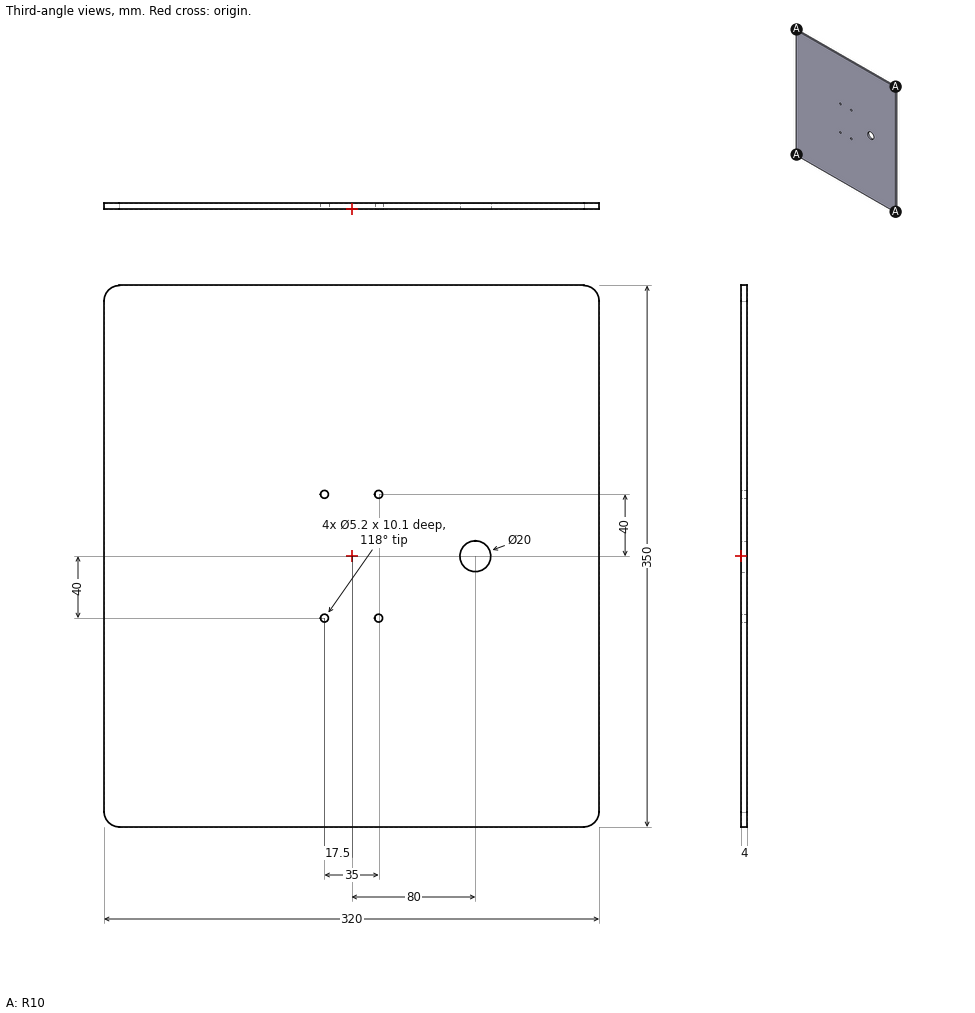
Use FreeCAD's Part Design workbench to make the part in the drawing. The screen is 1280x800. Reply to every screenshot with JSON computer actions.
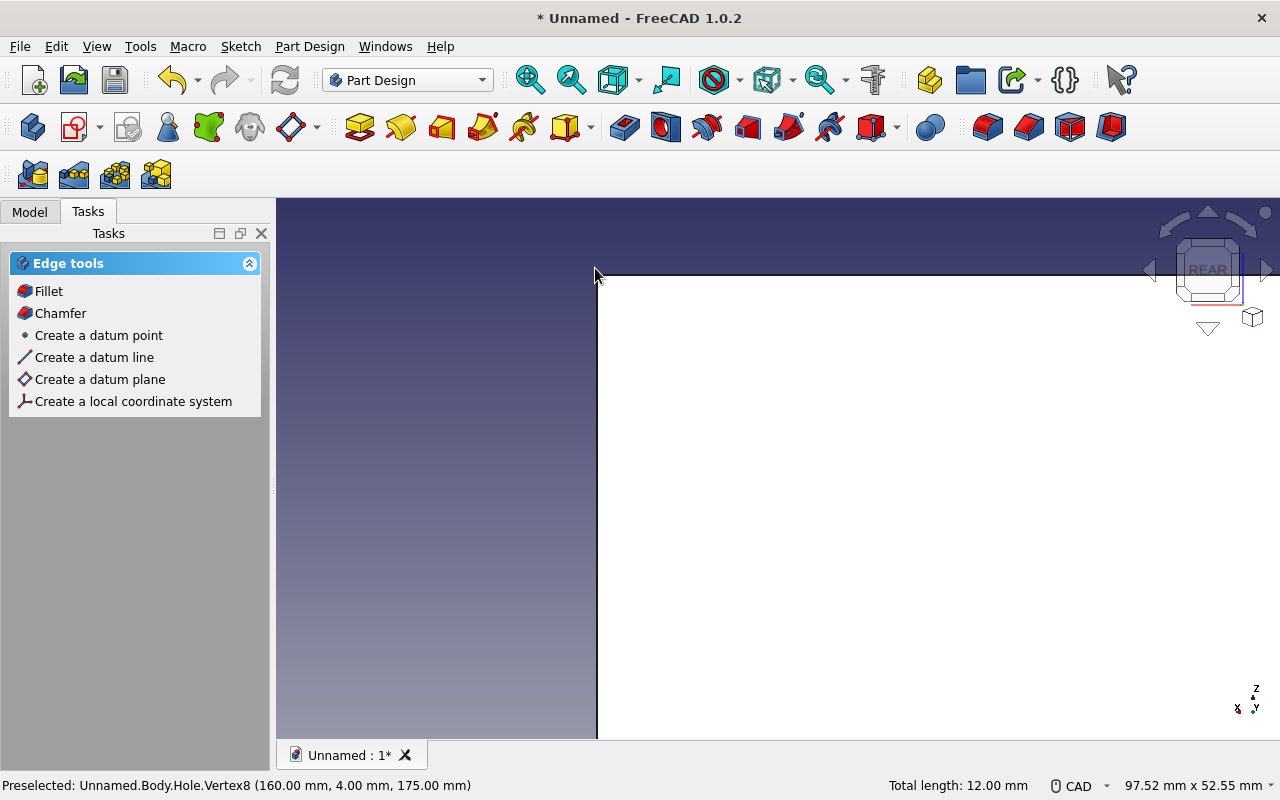
{"action": "key", "text": "v f"}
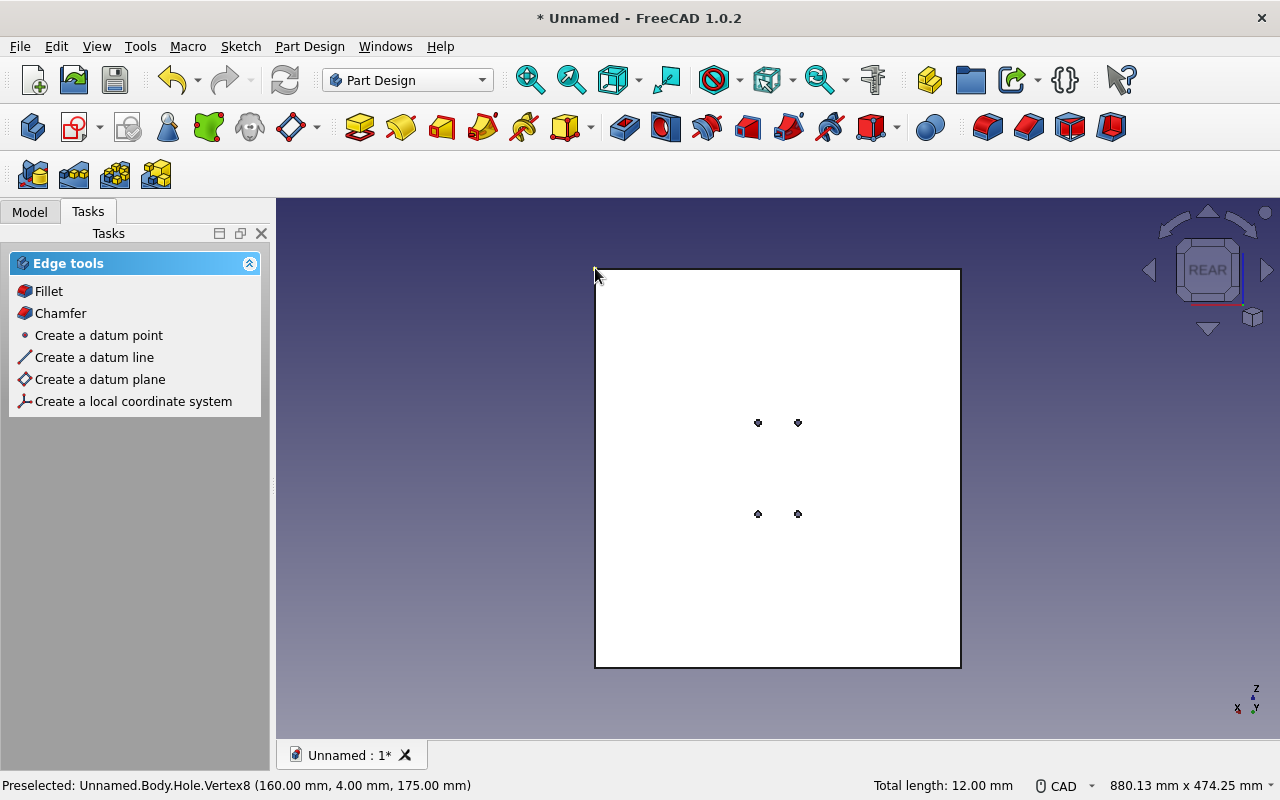
{"action": "key", "text": "6"}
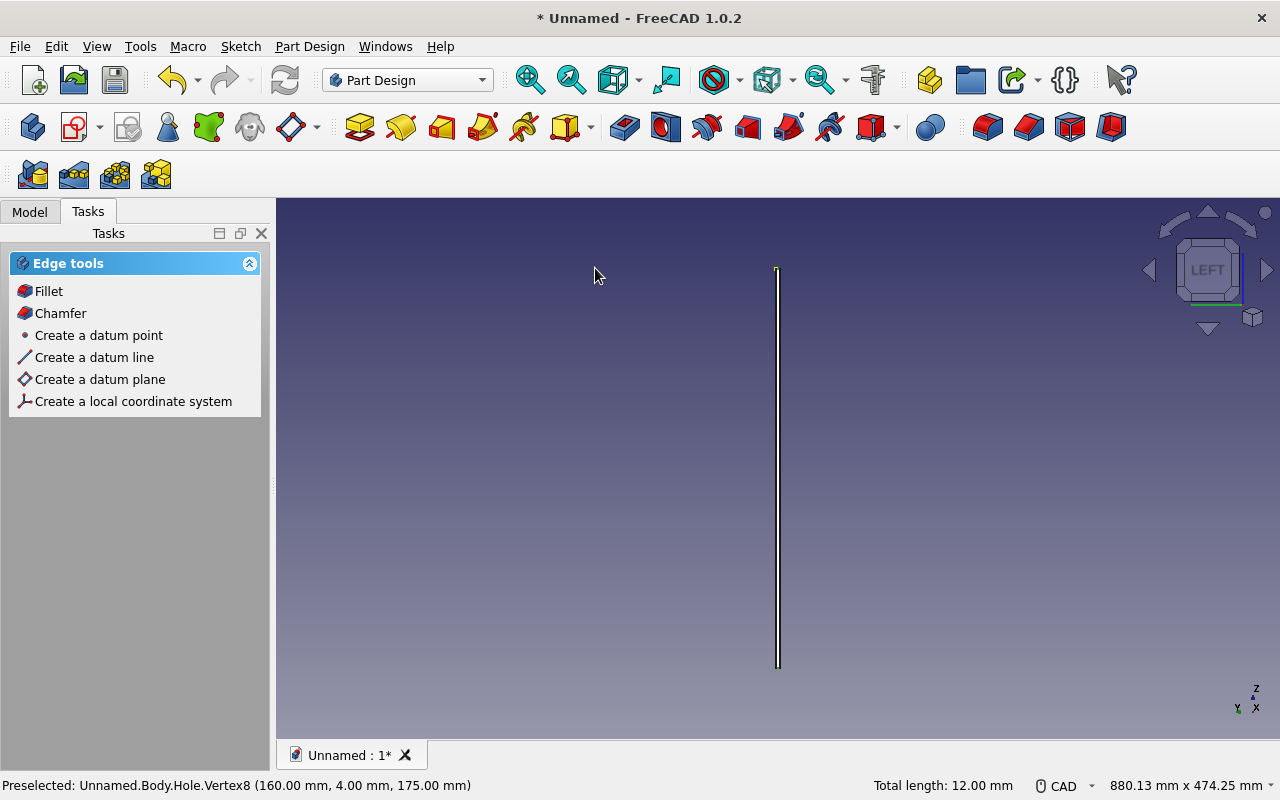
{"action": "scroll", "coordinate": [778, 268], "scroll_direction": "up", "scroll_amount": 11}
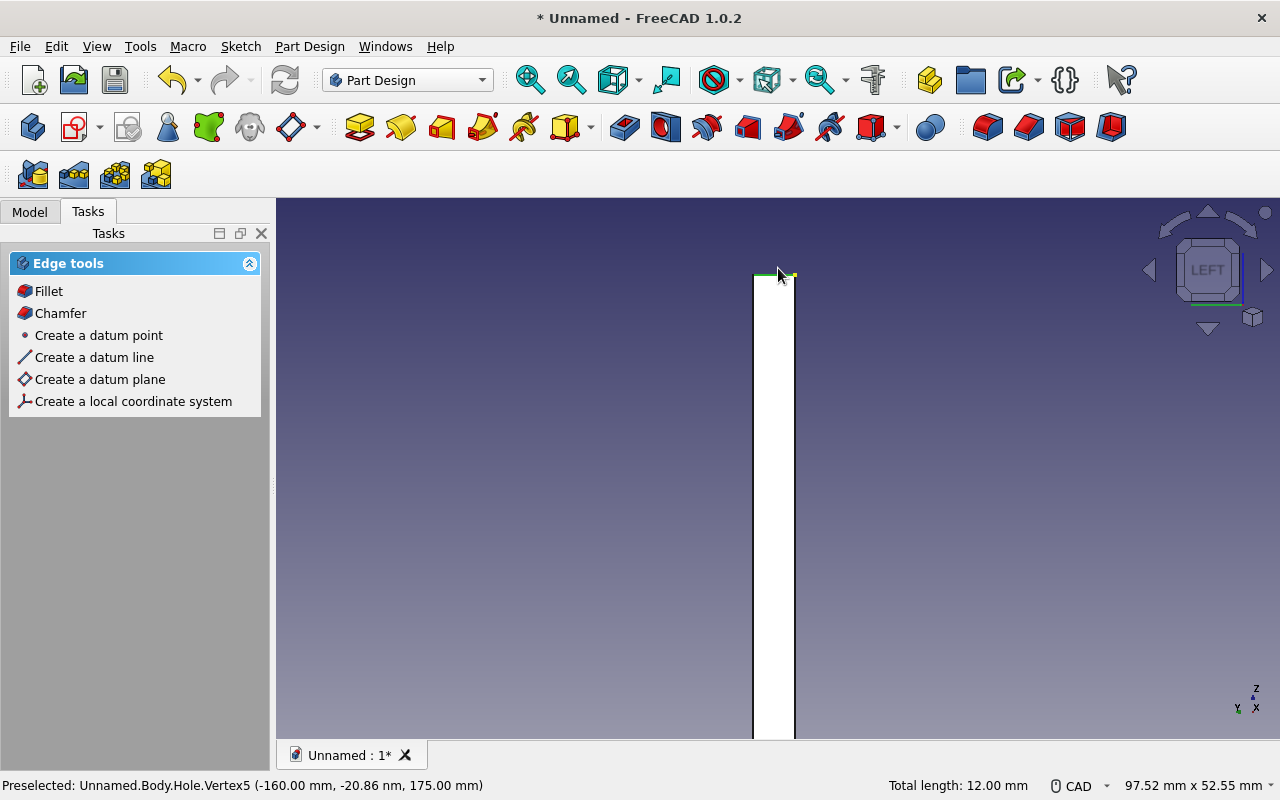
{"action": "left_click", "coordinate": [531, 80]}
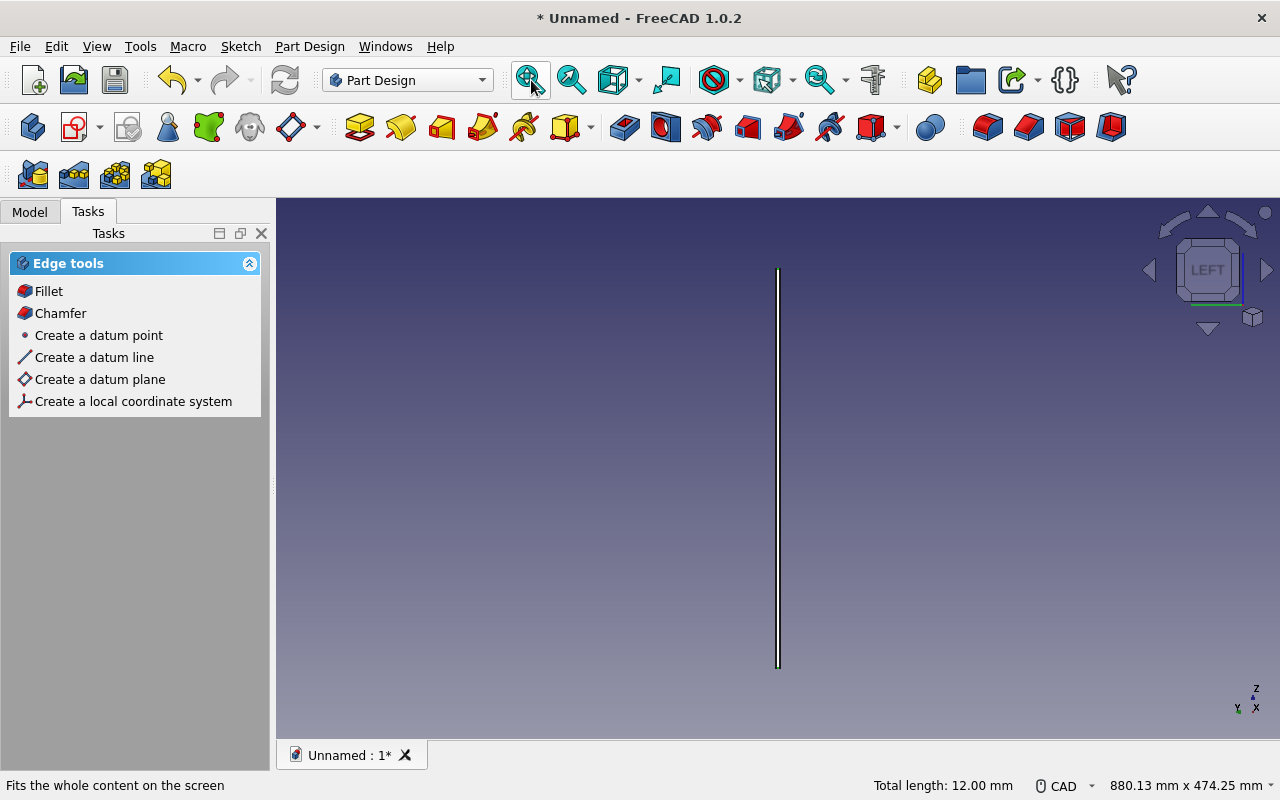
{"action": "key", "text": "v 3"}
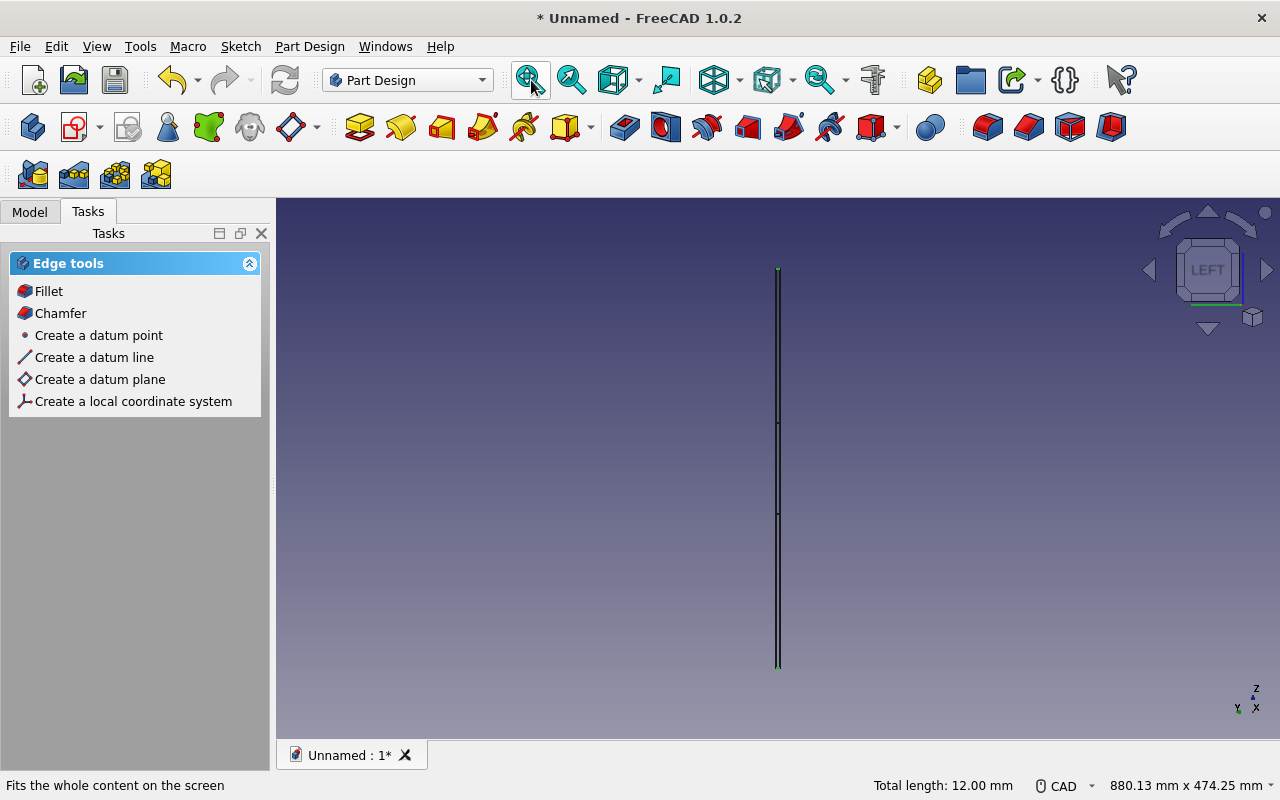
{"action": "key", "text": "0"}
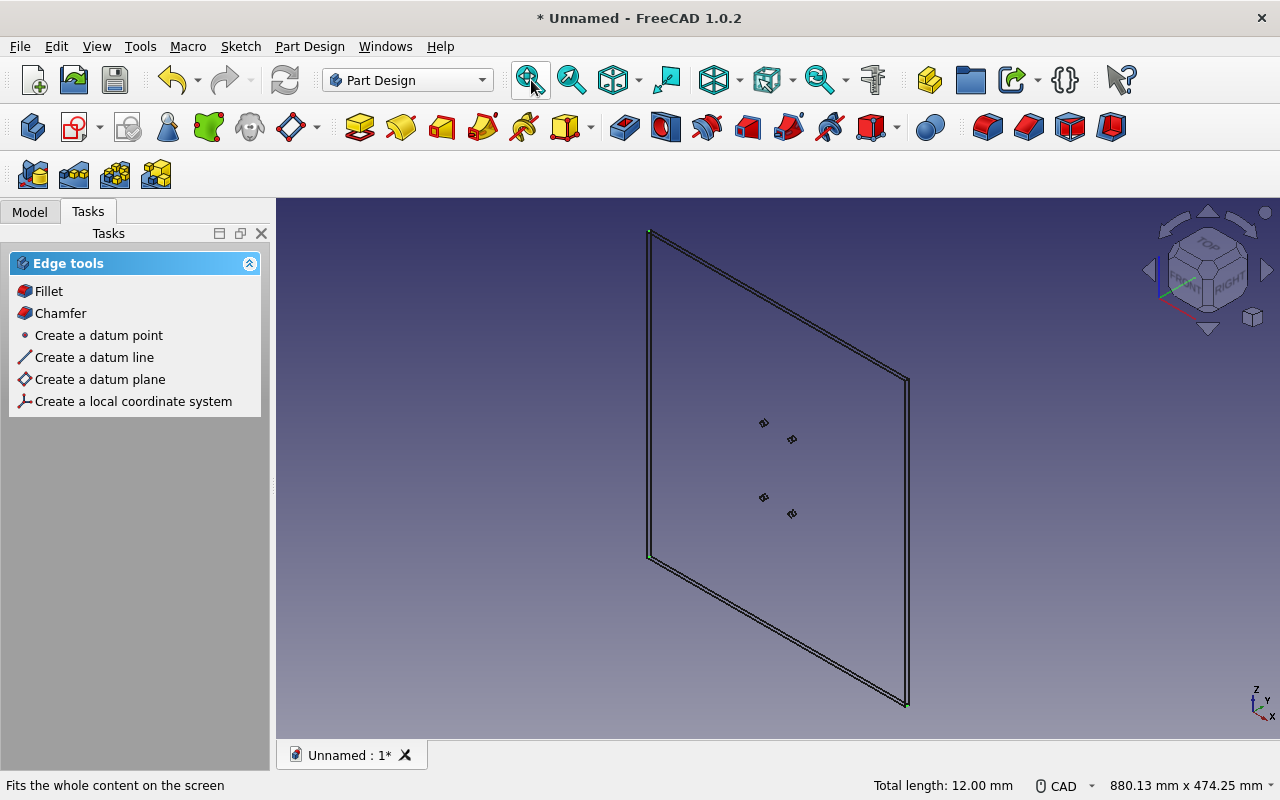
{"action": "scroll", "coordinate": [907, 379], "scroll_direction": "up", "scroll_amount": 11}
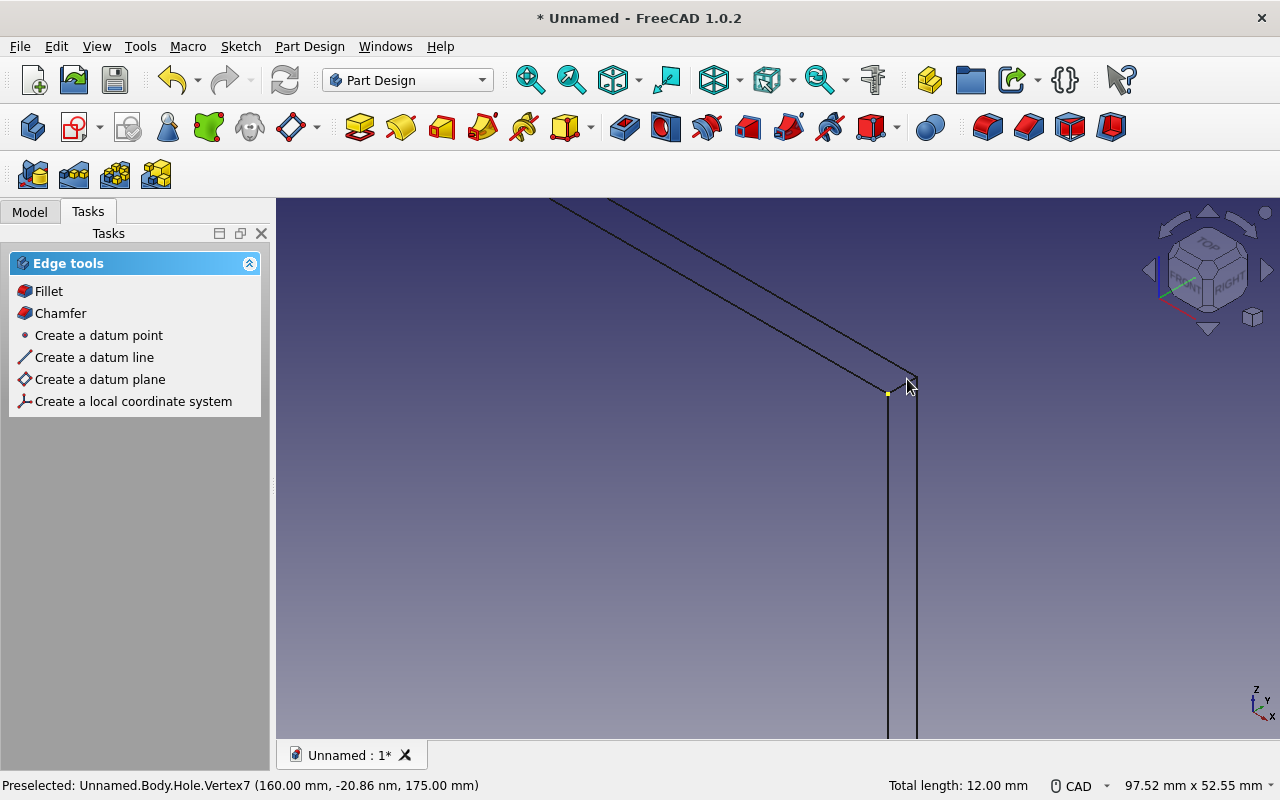
{"action": "left_click", "coordinate": [902, 384], "text": "ctrl"}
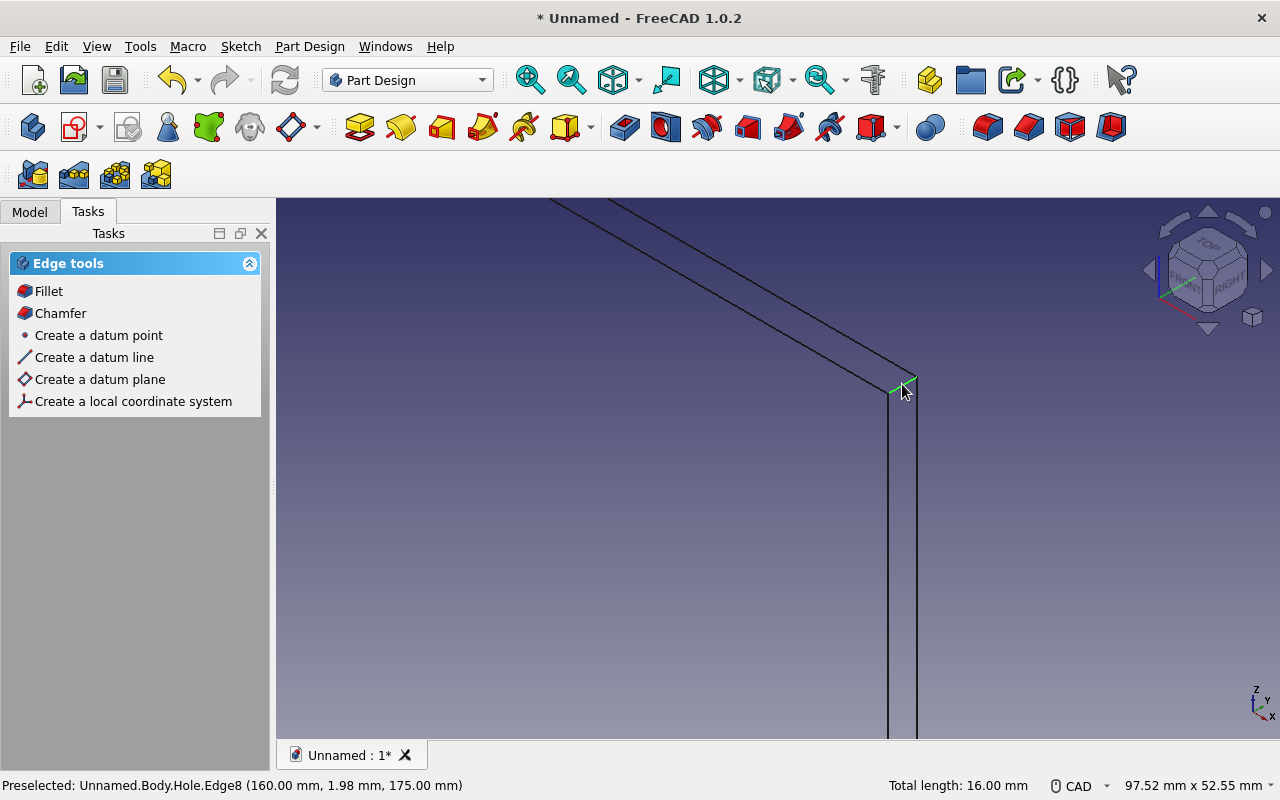
{"action": "key", "text": "v 1"}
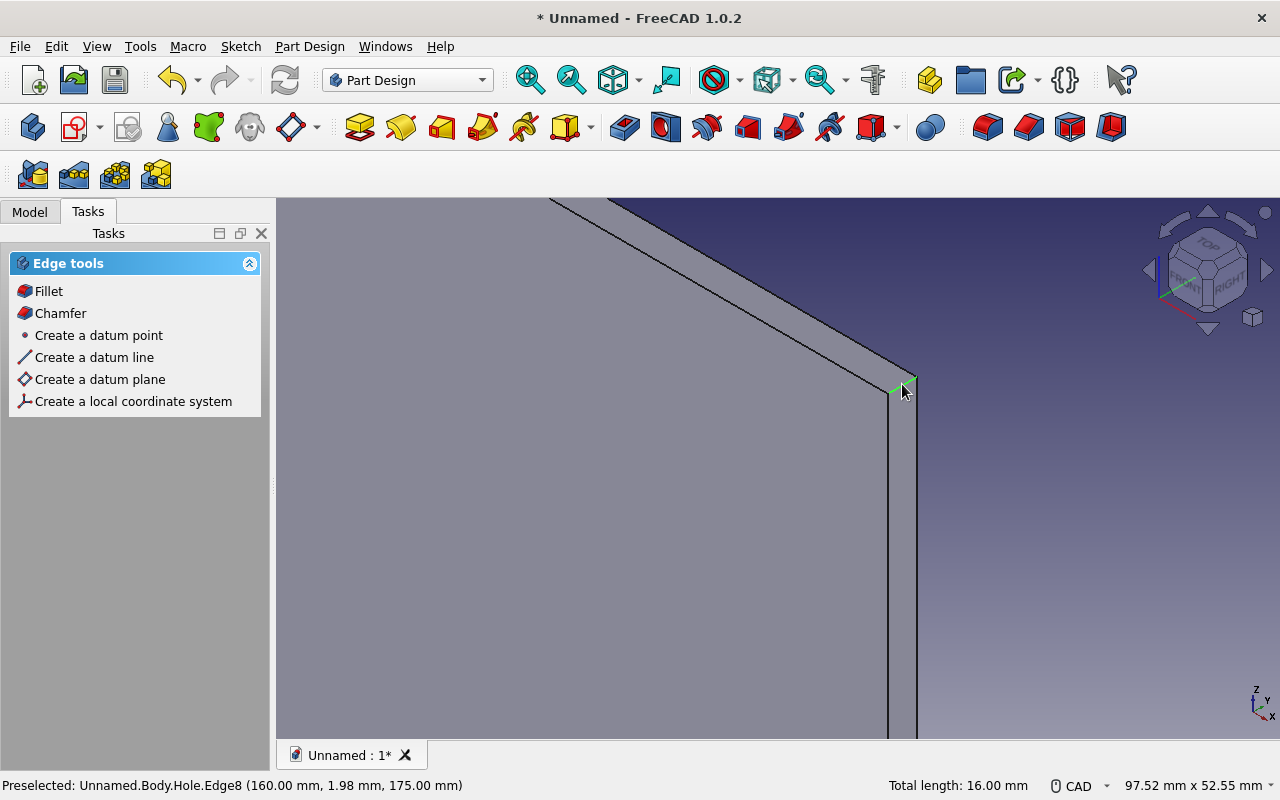
{"action": "left_click", "coordinate": [988, 128]}